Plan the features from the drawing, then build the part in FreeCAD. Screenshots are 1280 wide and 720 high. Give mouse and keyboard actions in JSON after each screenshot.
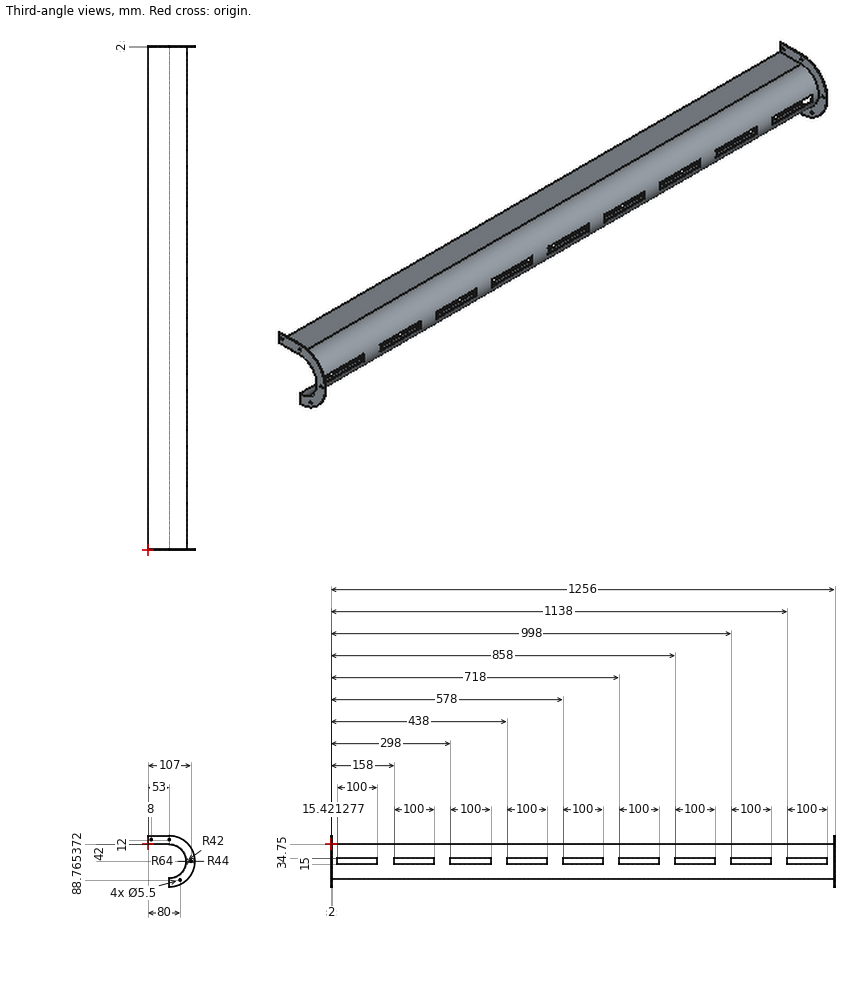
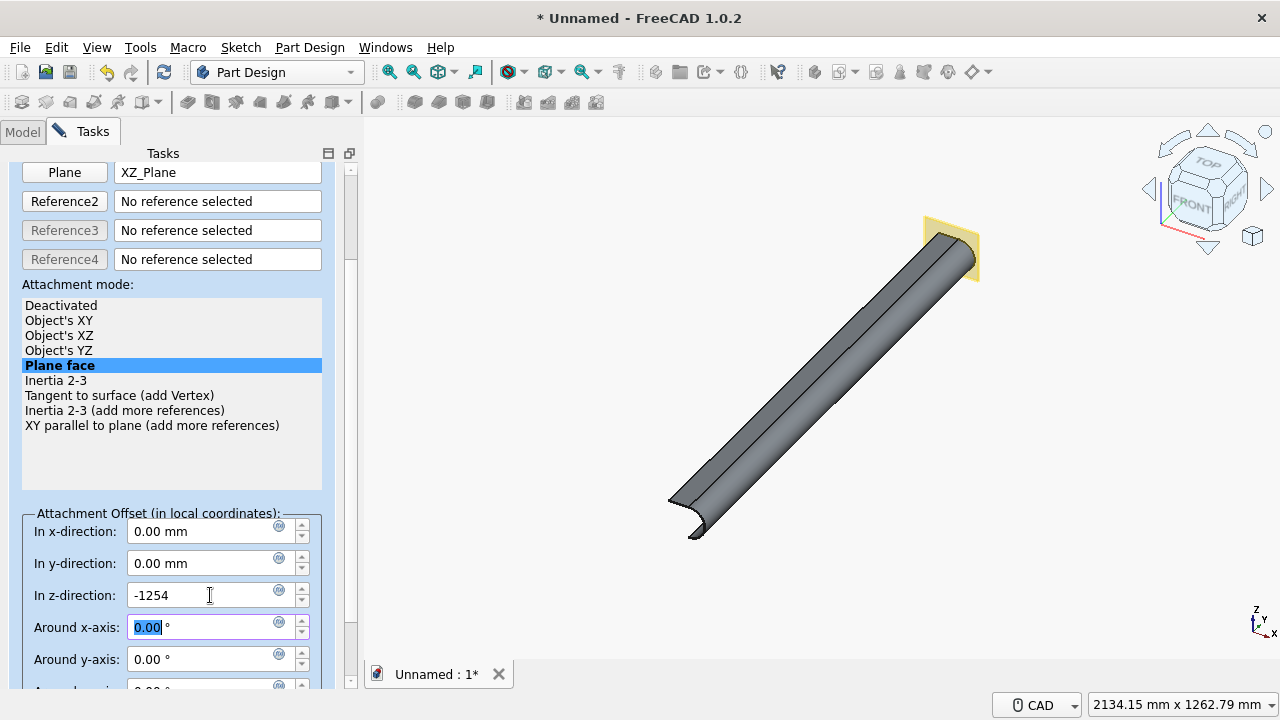
{"action": "scroll", "coordinate": [351, 426], "scroll_direction": "up", "scroll_amount": 3}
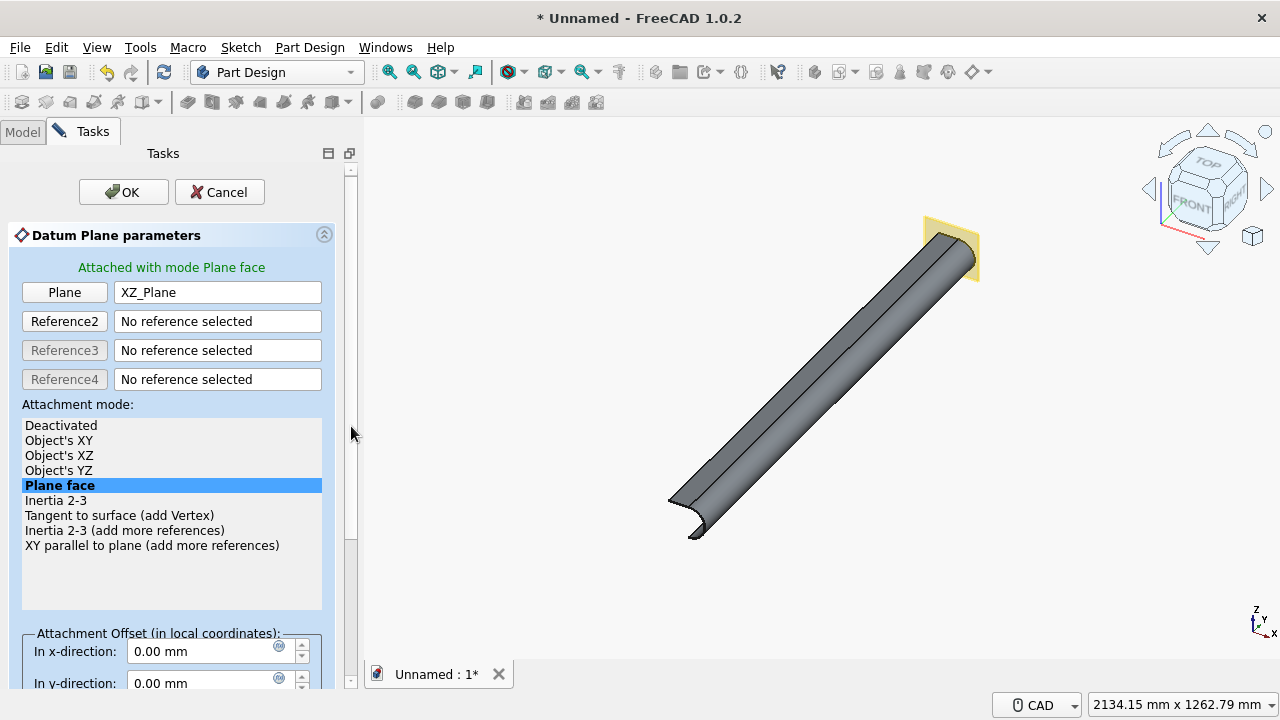
{"action": "left_click", "coordinate": [124, 192]}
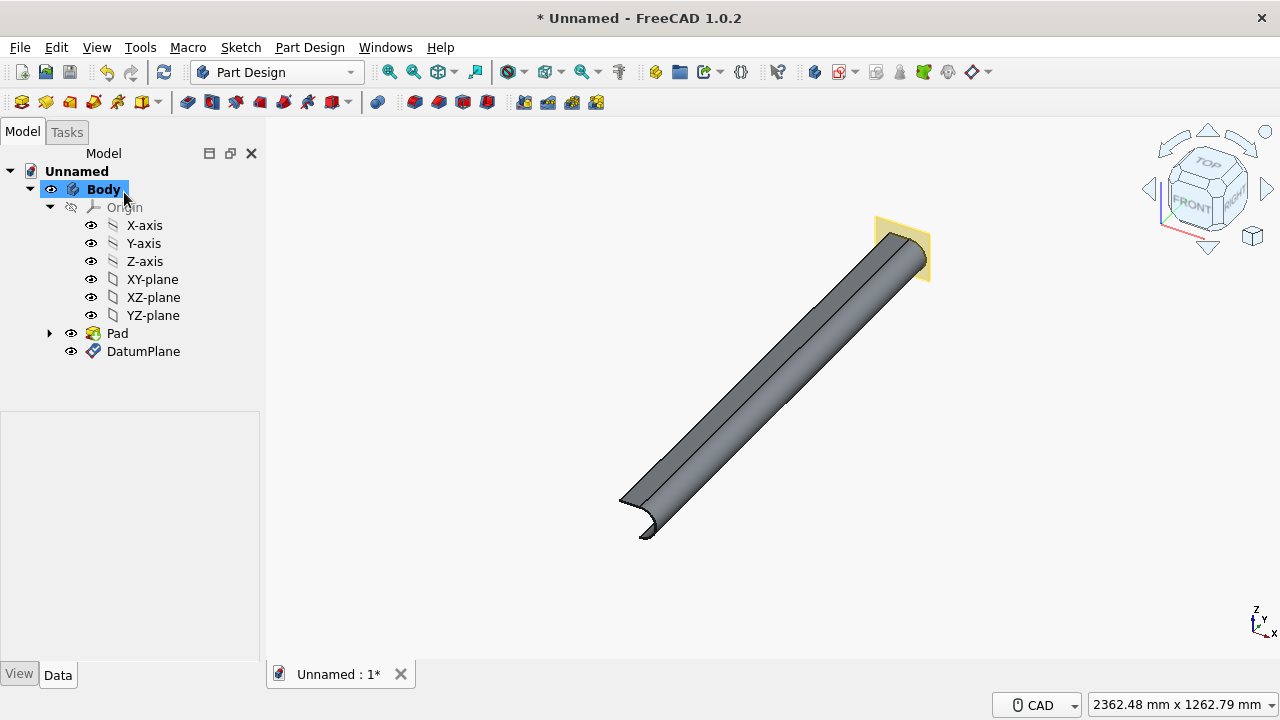
{"action": "left_click", "coordinate": [116, 351]}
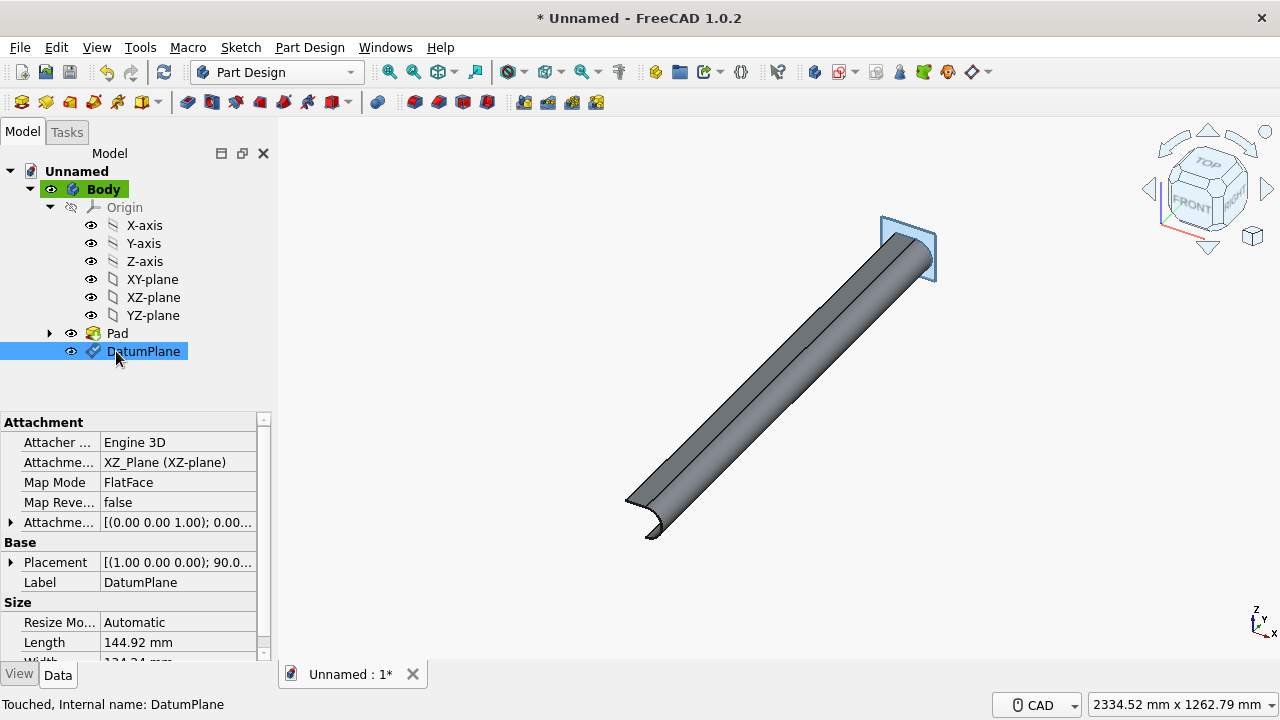
{"action": "left_click", "coordinate": [840, 72]}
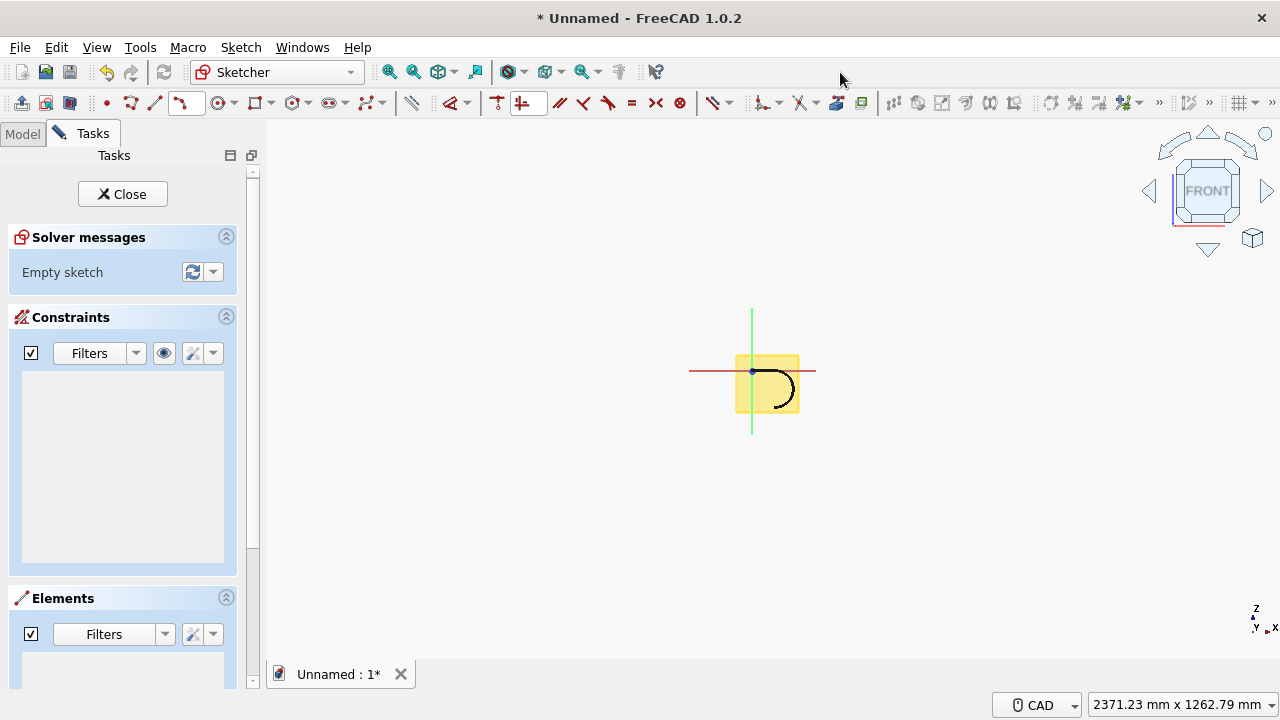
{"action": "left_click", "coordinate": [70, 104]}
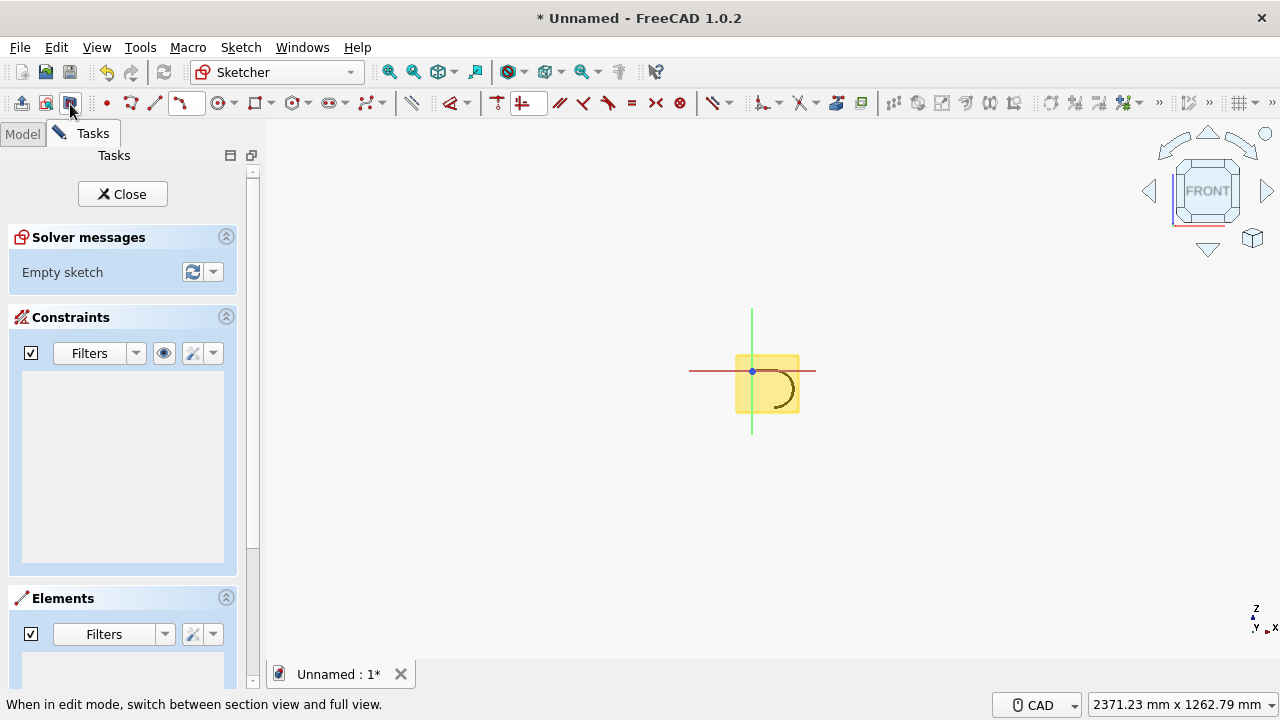
{"action": "scroll", "coordinate": [792, 389], "scroll_direction": "up", "scroll_amount": 9}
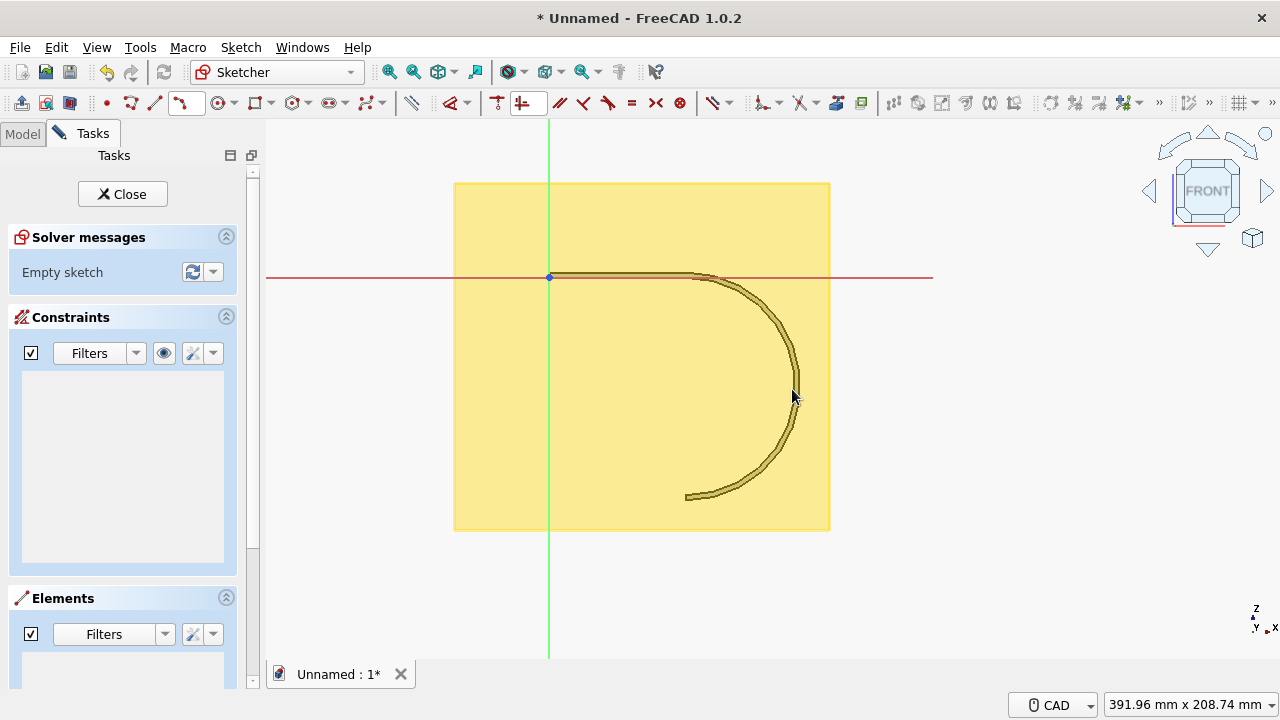
{"action": "left_click", "coordinate": [132, 104]}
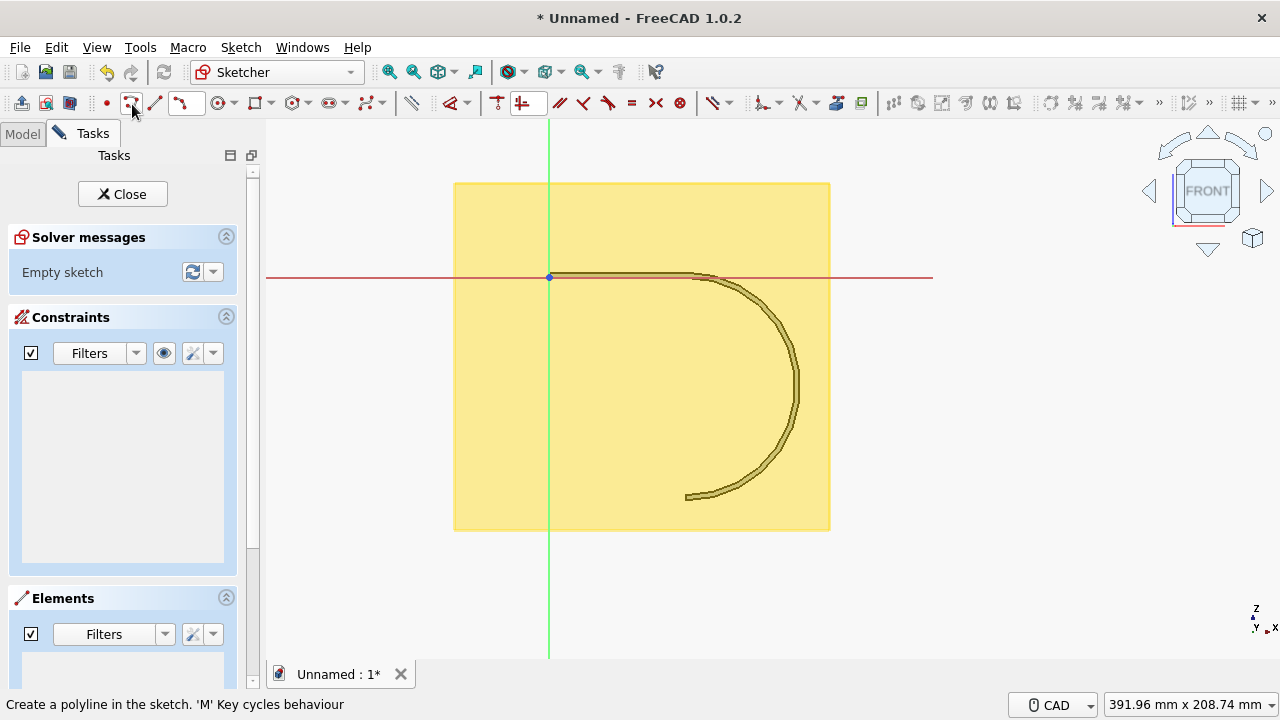
{"action": "left_click", "coordinate": [686, 278]}
{"action": "left_click", "coordinate": [549, 278]}
{"action": "left_click", "coordinate": [558, 221]}
{"action": "left_click", "coordinate": [686, 221]}
{"action": "right_click", "coordinate": [686, 221]}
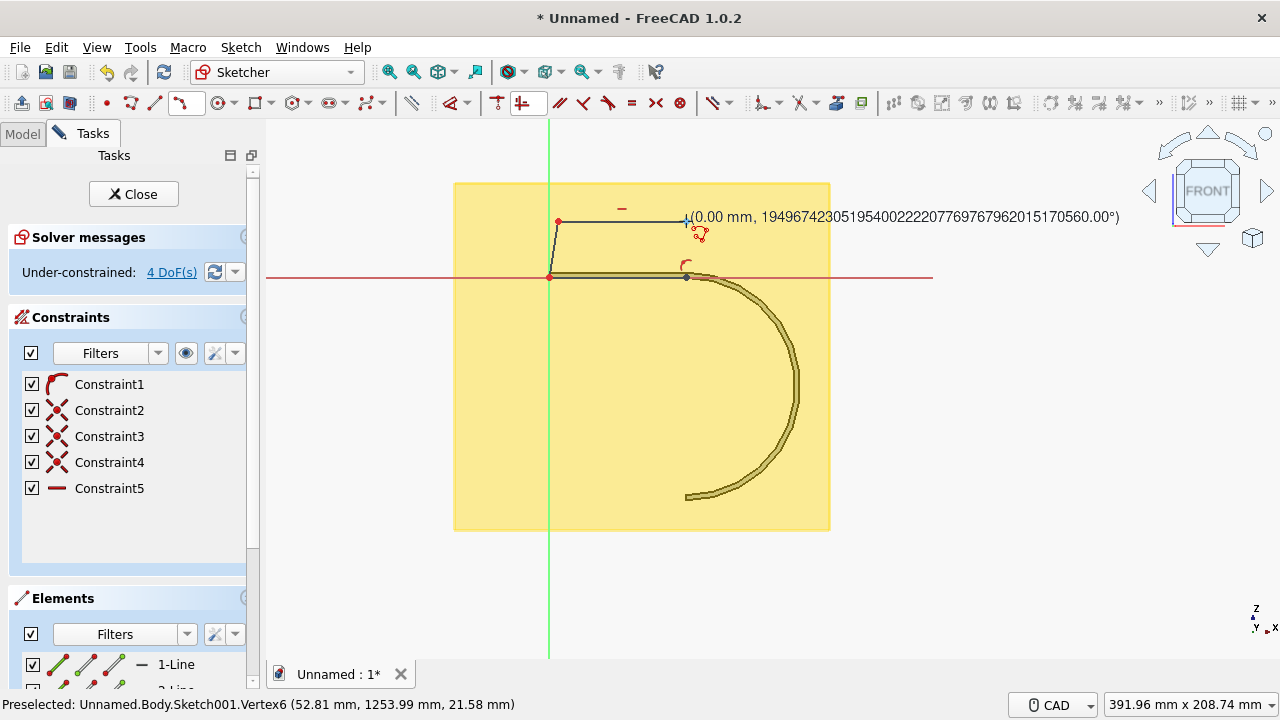
{"action": "left_click", "coordinate": [156, 104]}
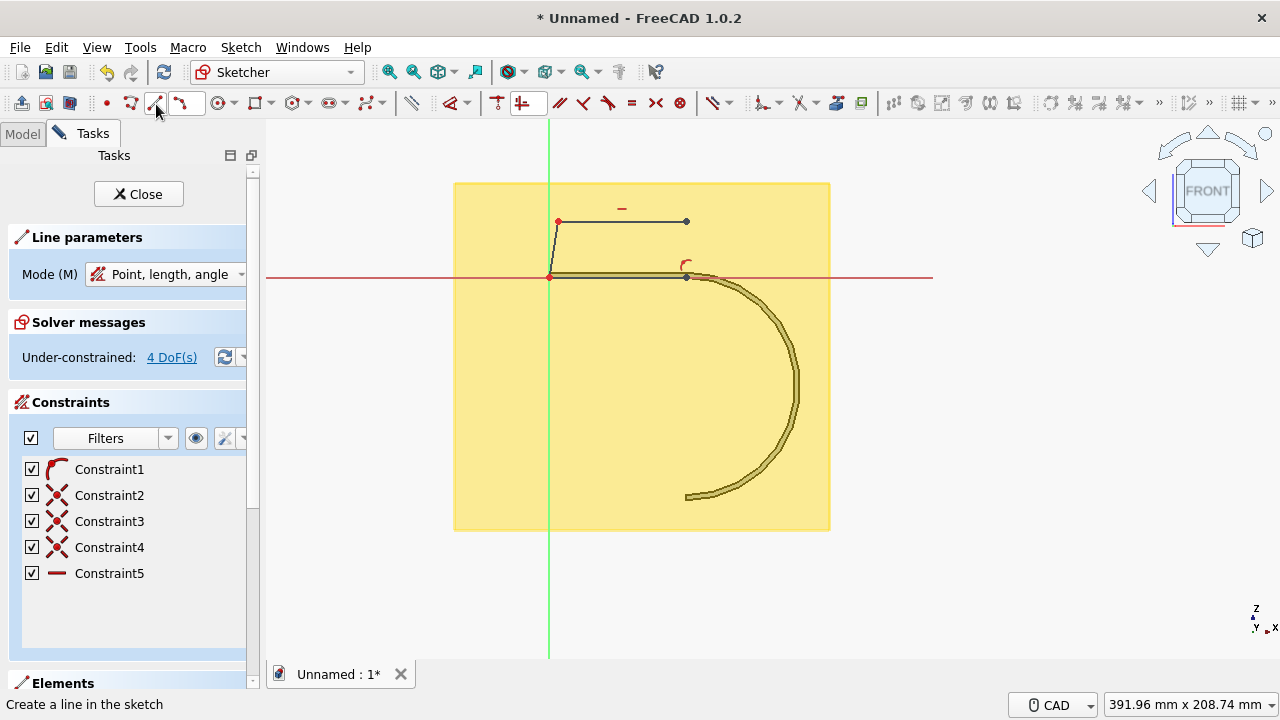
{"action": "left_click", "coordinate": [686, 552]}
{"action": "left_click", "coordinate": [686, 495]}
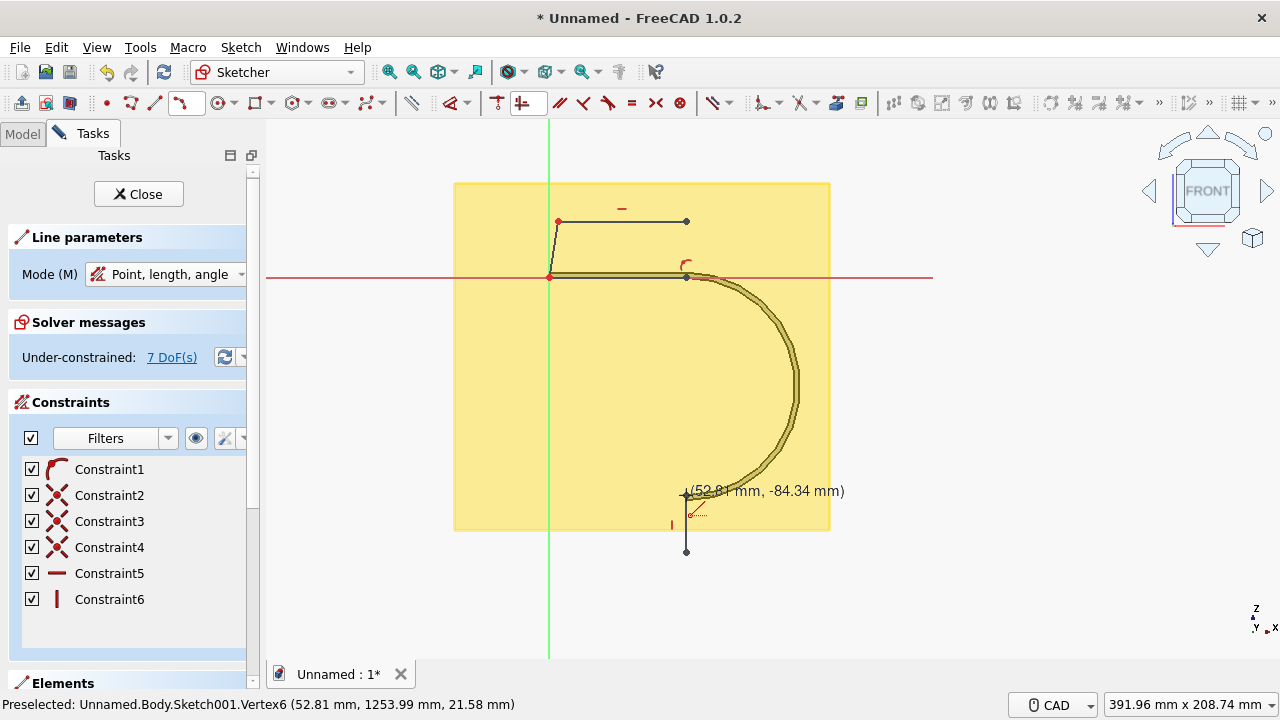
{"action": "left_click", "coordinate": [180, 104]}